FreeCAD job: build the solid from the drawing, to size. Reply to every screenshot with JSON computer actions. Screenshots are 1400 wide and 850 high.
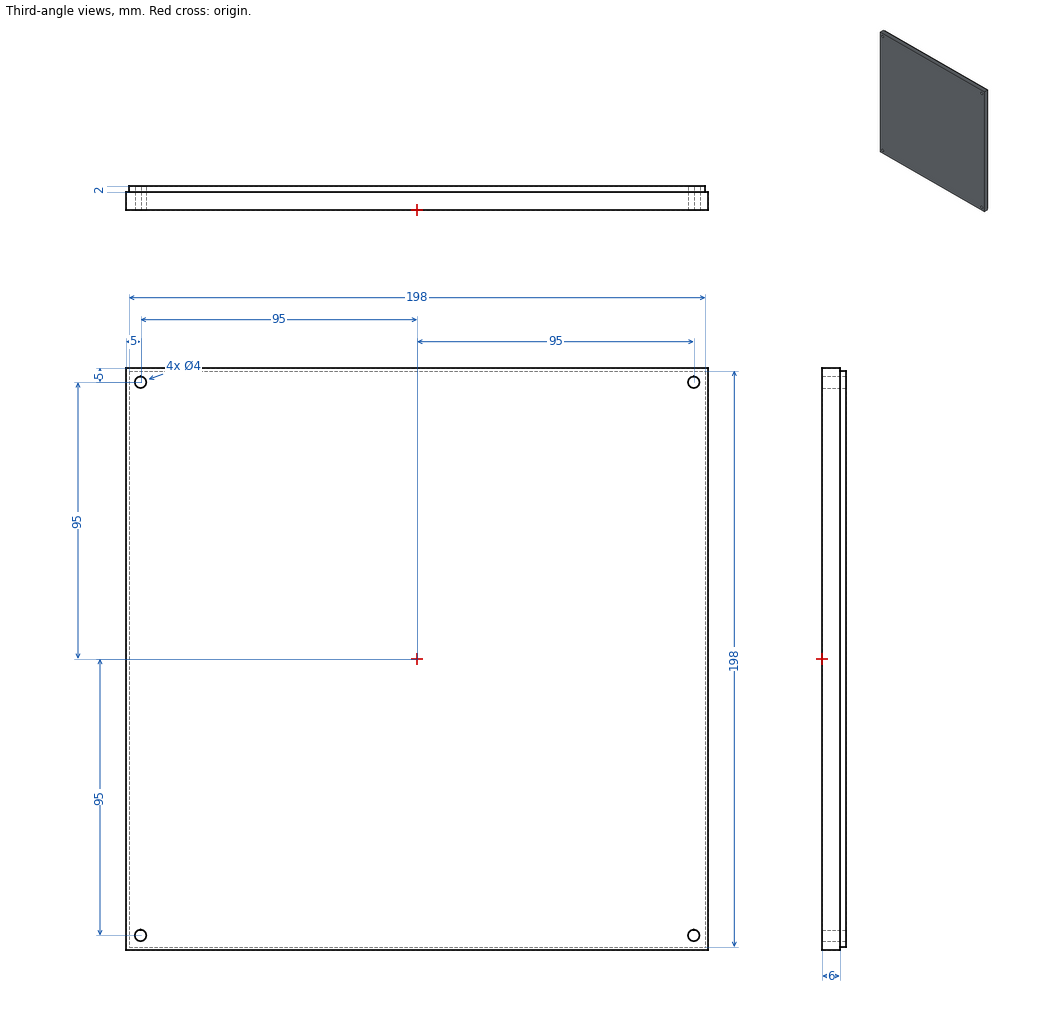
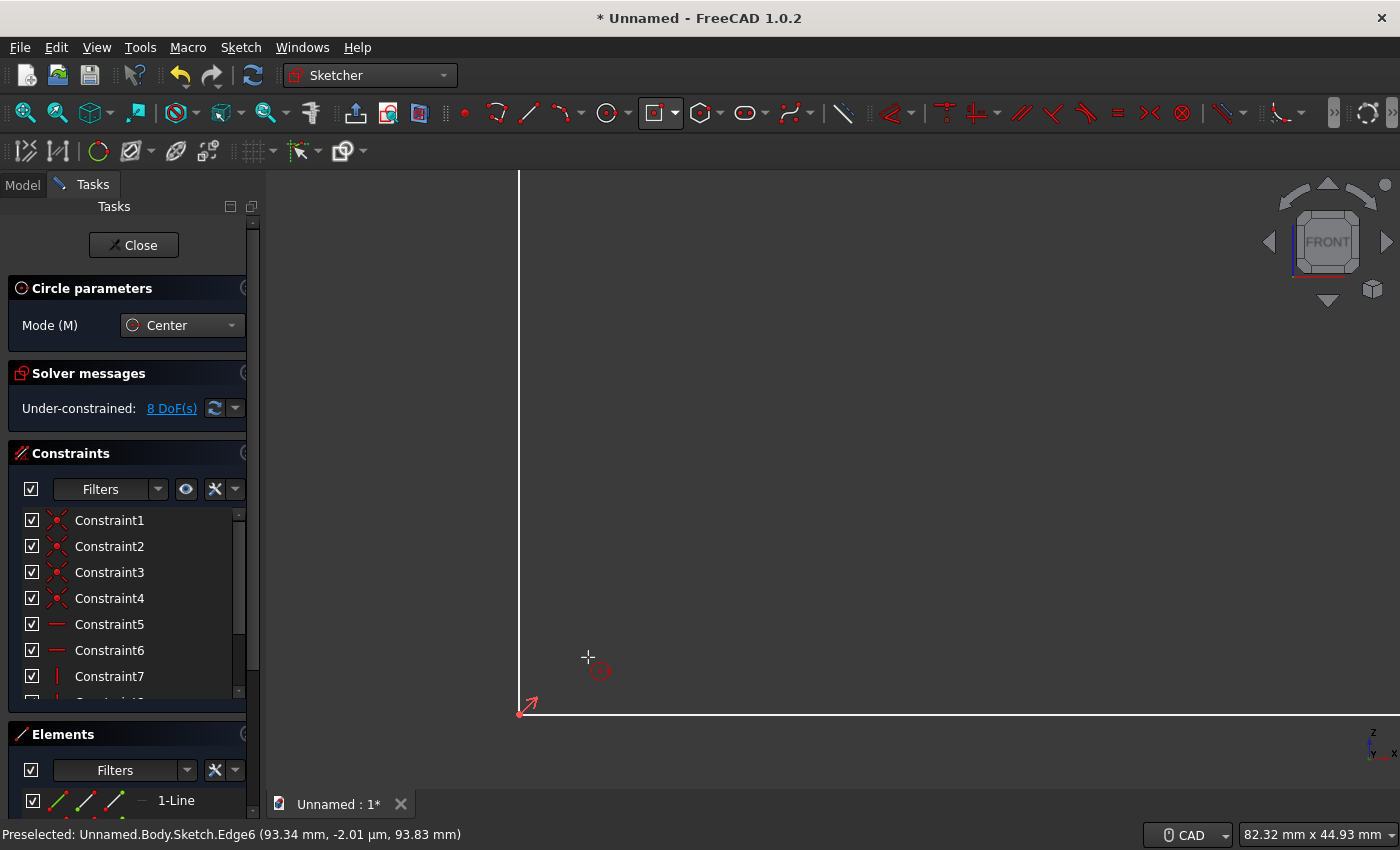
{"action": "scroll", "coordinate": [588, 657], "scroll_direction": "down", "scroll_amount": 10}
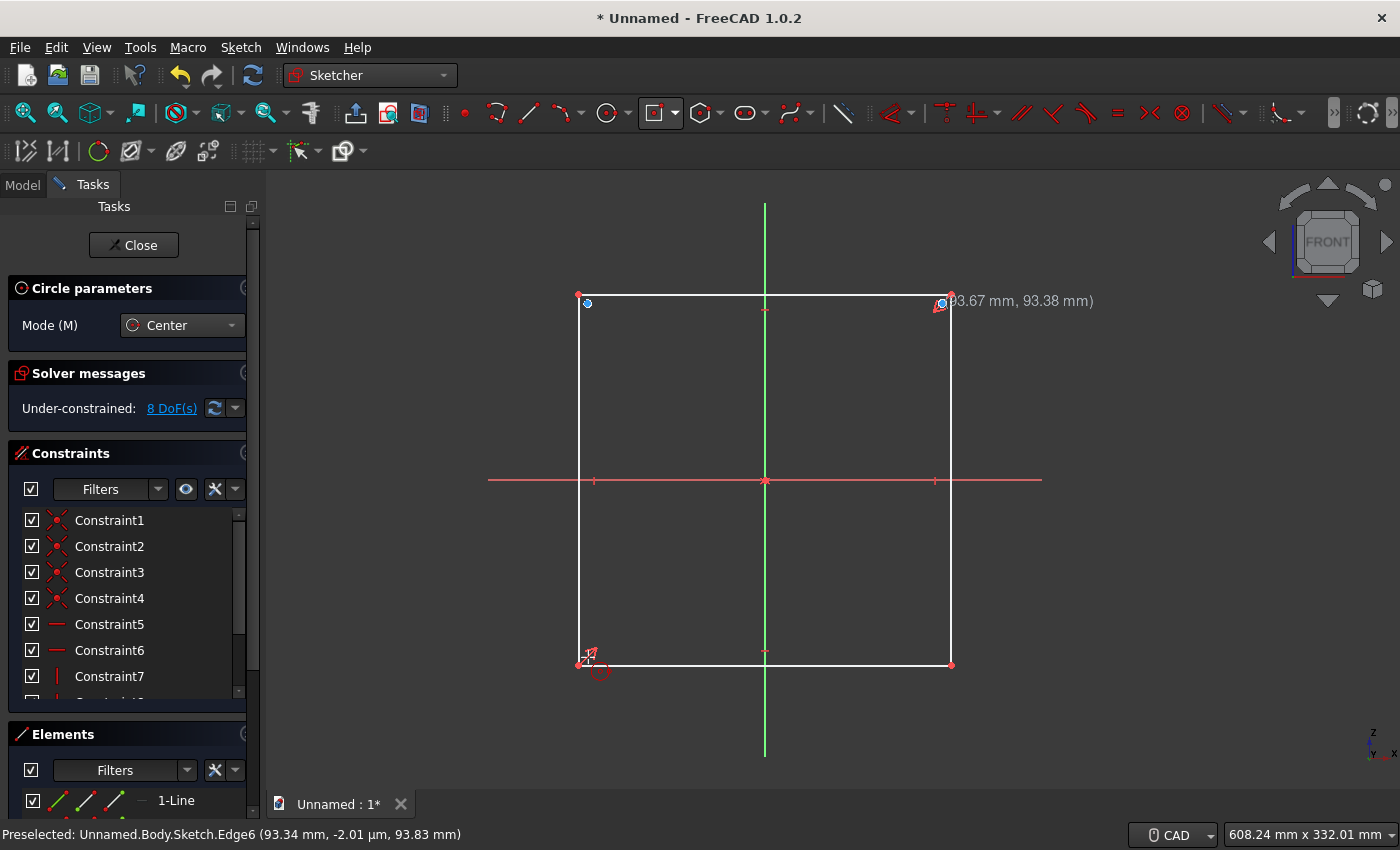
{"action": "scroll", "coordinate": [588, 657], "scroll_direction": "up", "scroll_amount": 3}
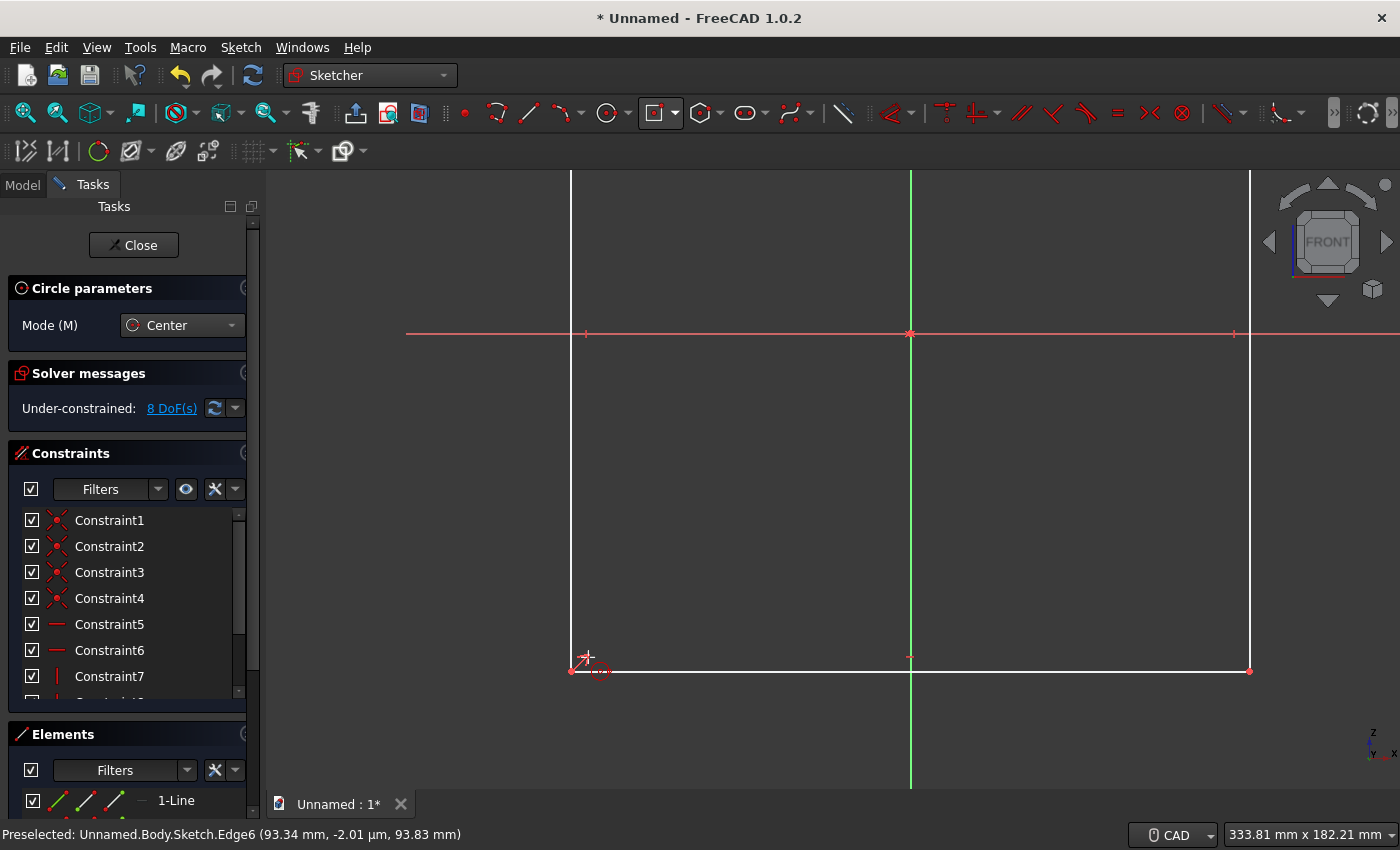
{"action": "left_click", "coordinate": [588, 657]}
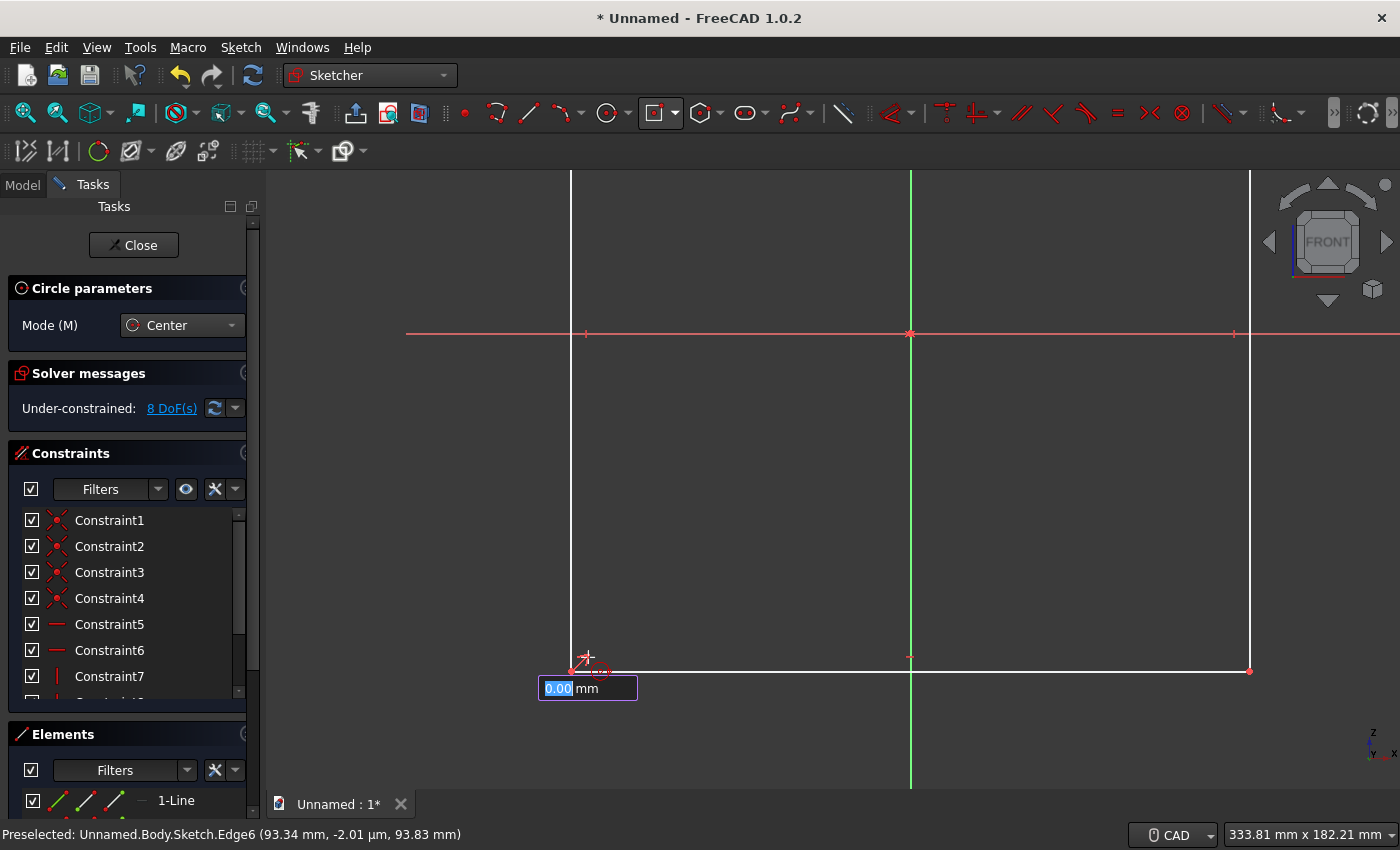
{"action": "scroll", "coordinate": [593, 652], "scroll_direction": "up", "scroll_amount": 5}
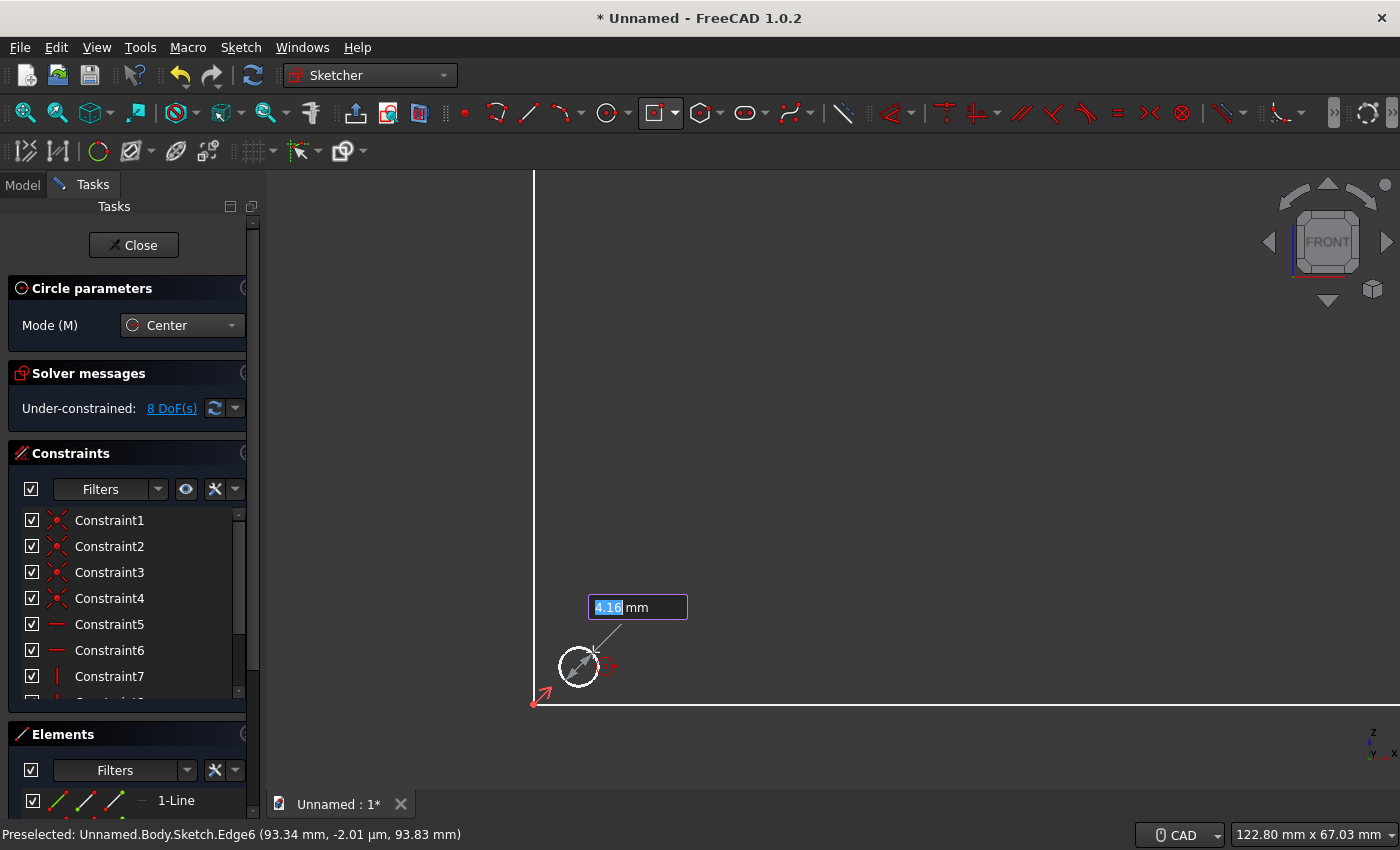
{"action": "left_click", "coordinate": [592, 650]}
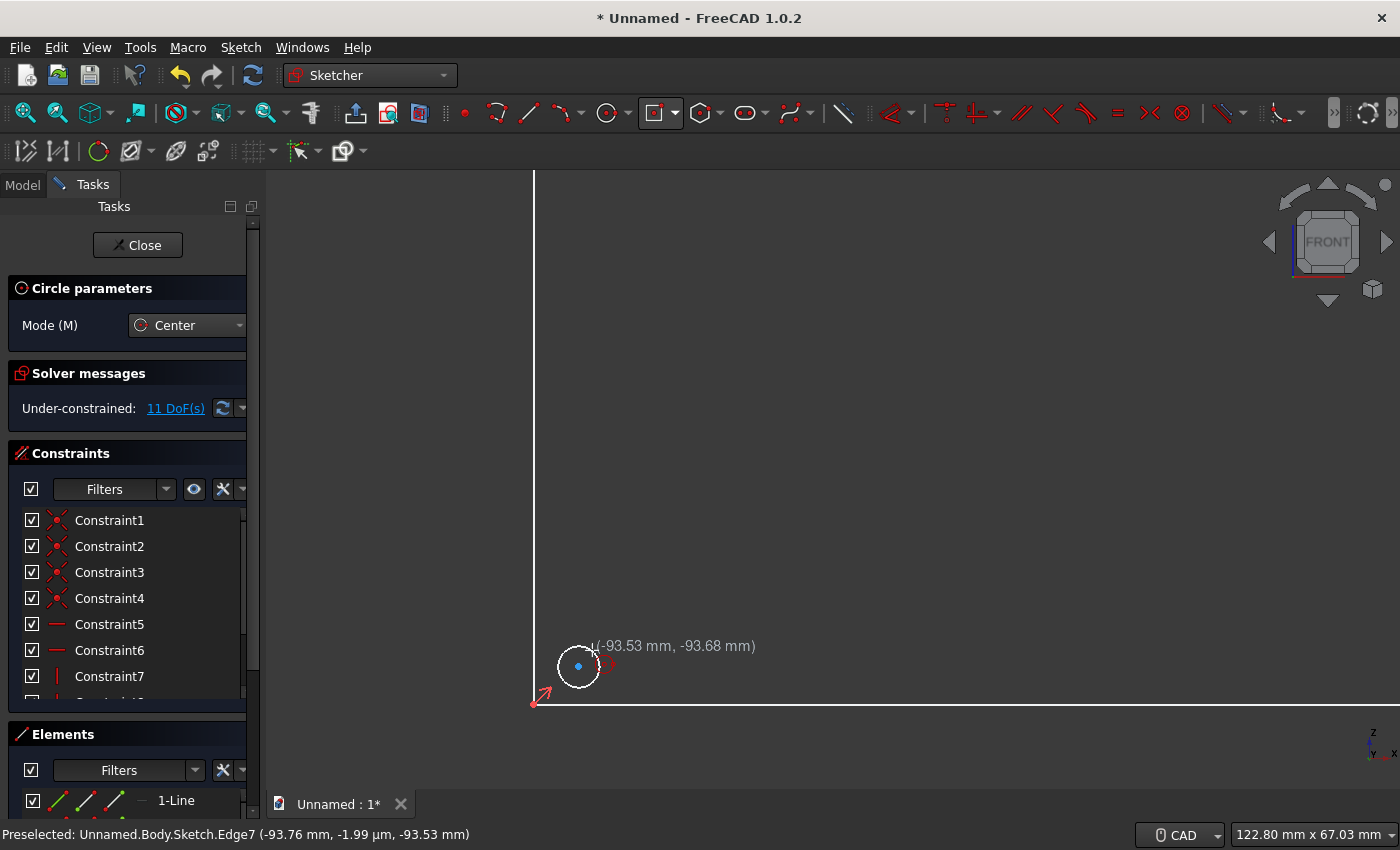
{"action": "scroll", "coordinate": [590, 655], "scroll_direction": "down", "scroll_amount": 8}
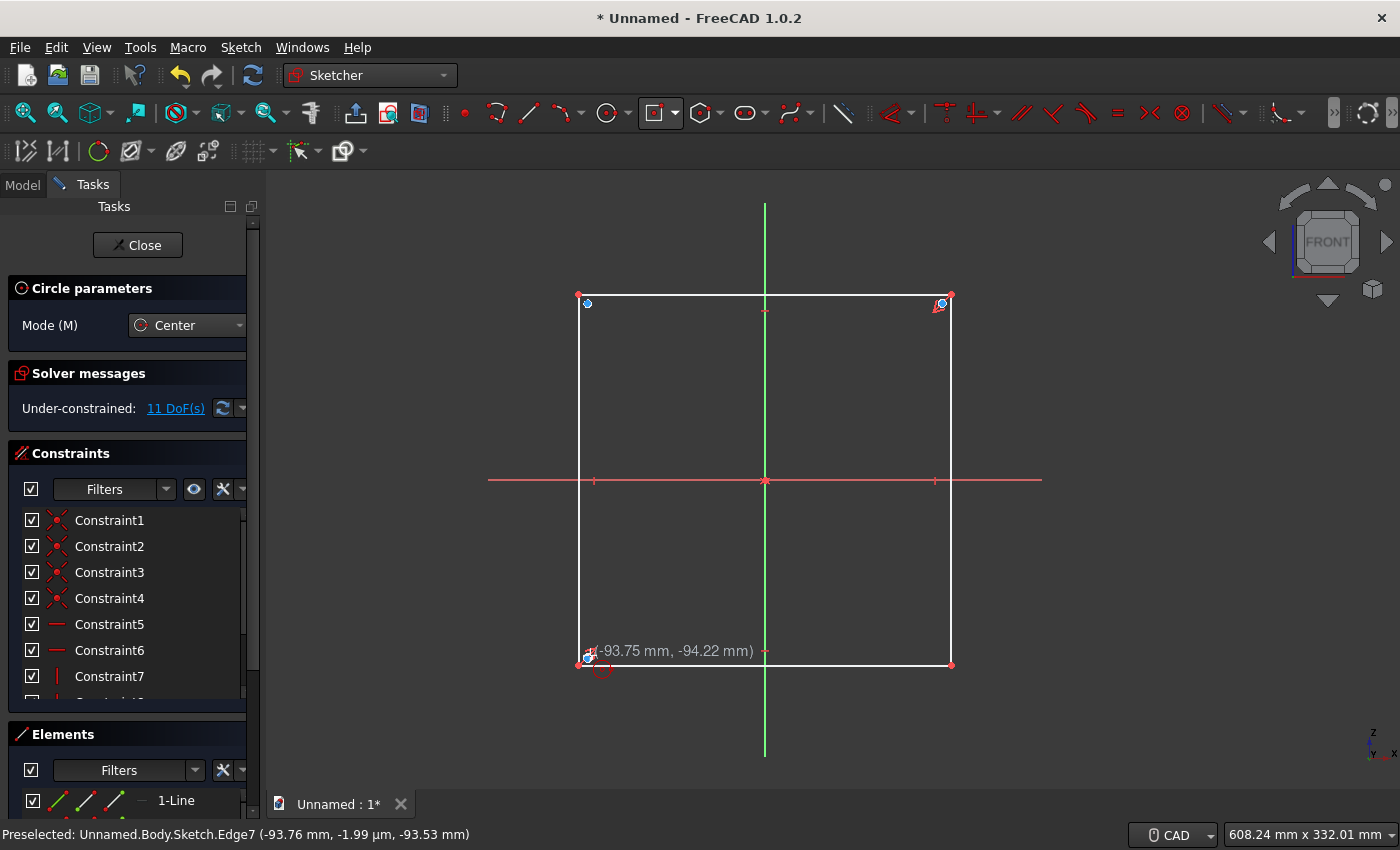
{"action": "scroll", "coordinate": [942, 657], "scroll_direction": "up", "scroll_amount": 10}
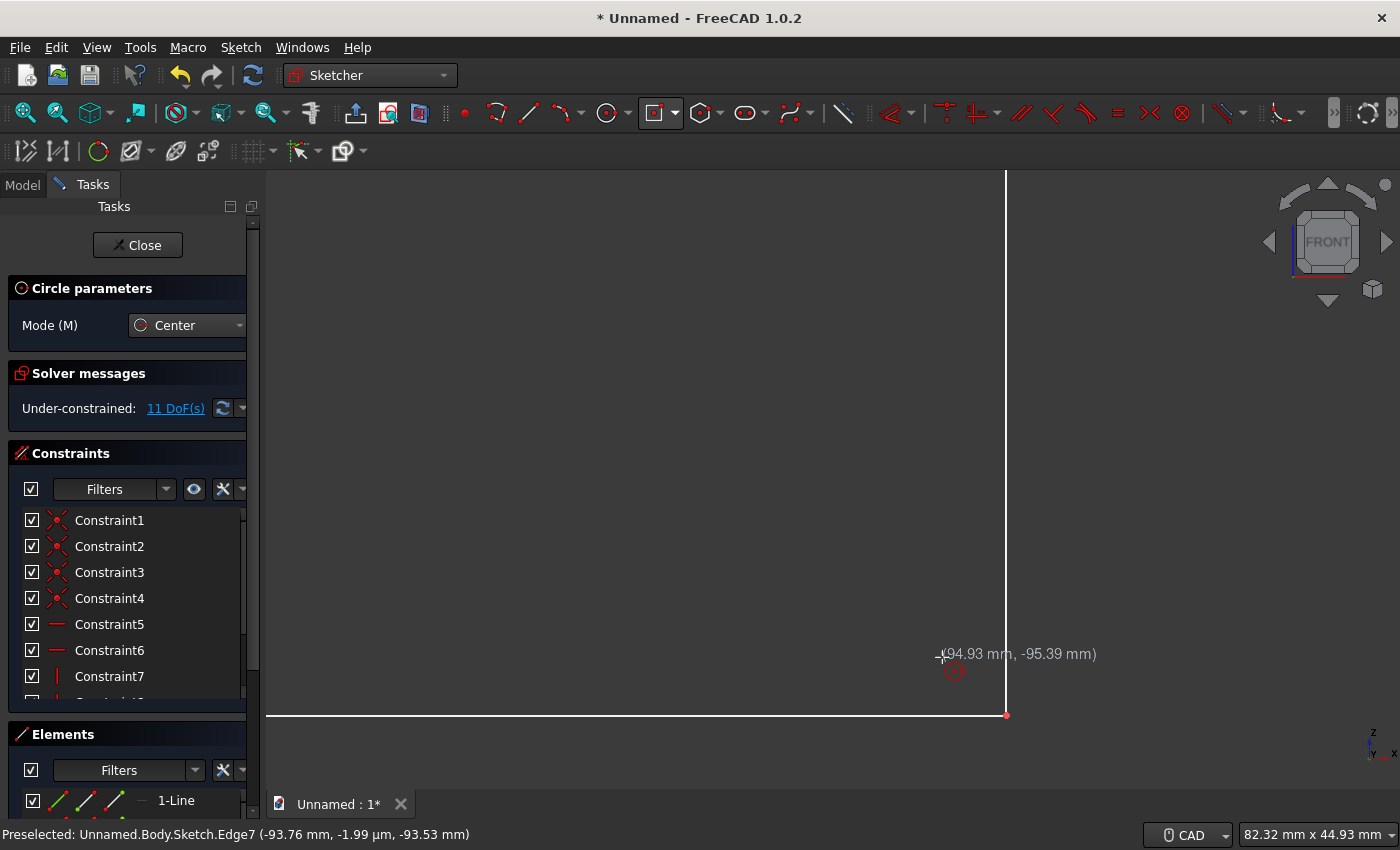
{"action": "scroll", "coordinate": [942, 657], "scroll_direction": "down", "scroll_amount": 10}